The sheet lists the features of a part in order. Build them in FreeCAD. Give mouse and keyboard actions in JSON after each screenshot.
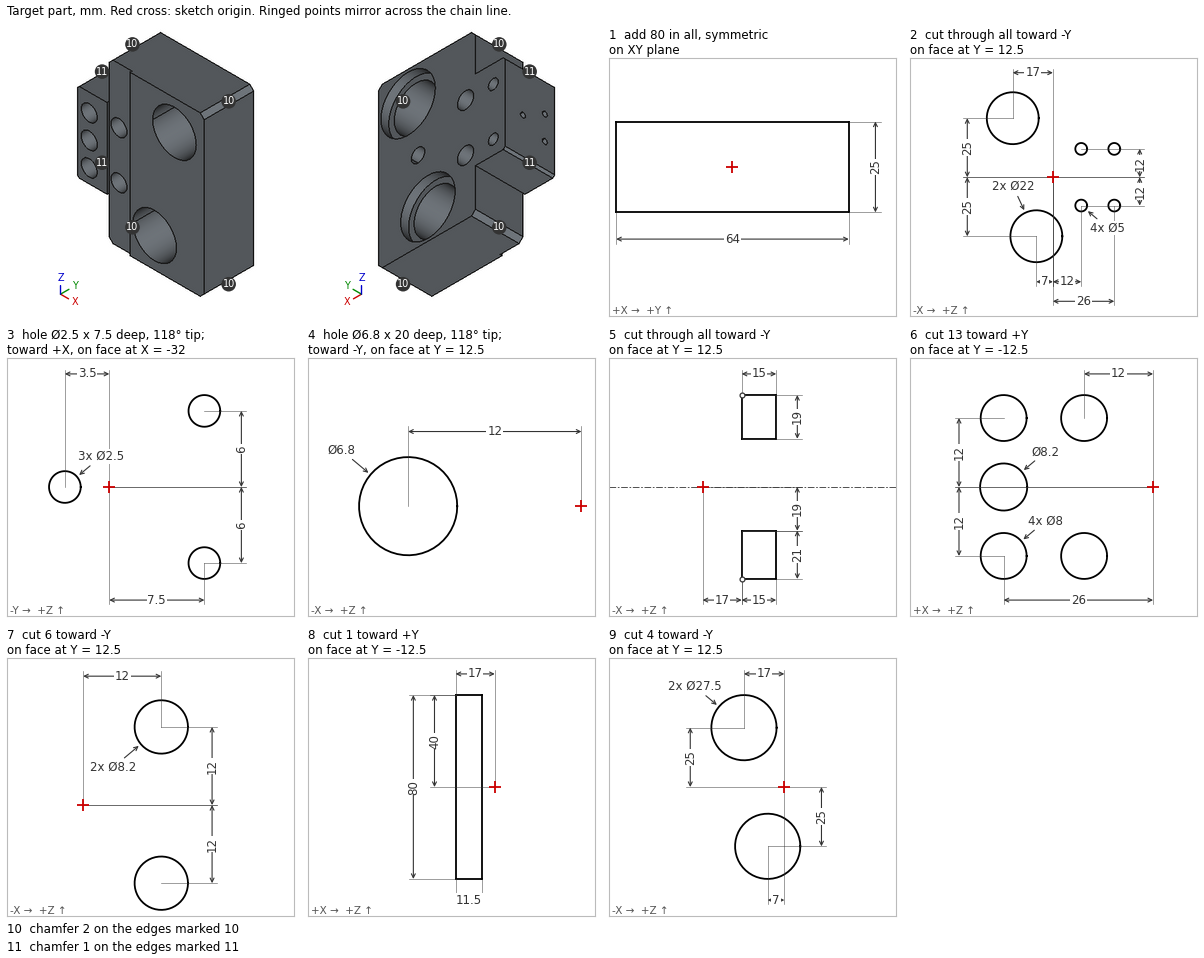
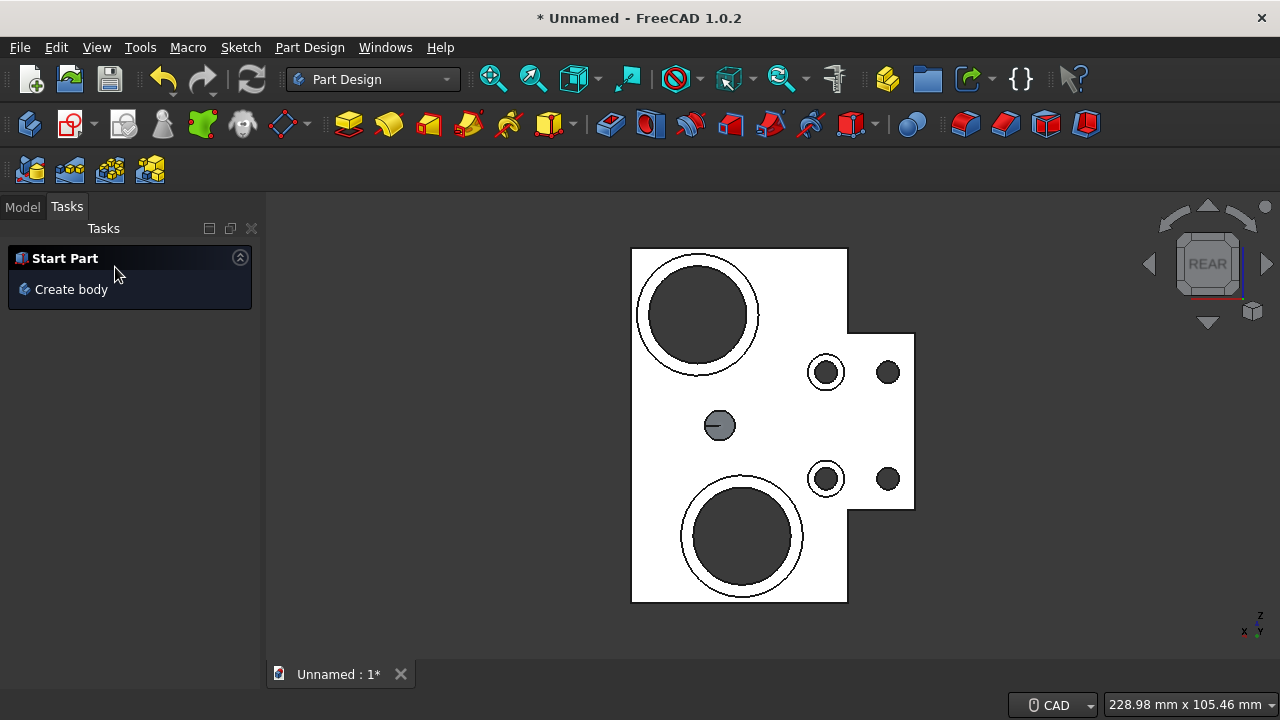
{"action": "key", "text": "0"}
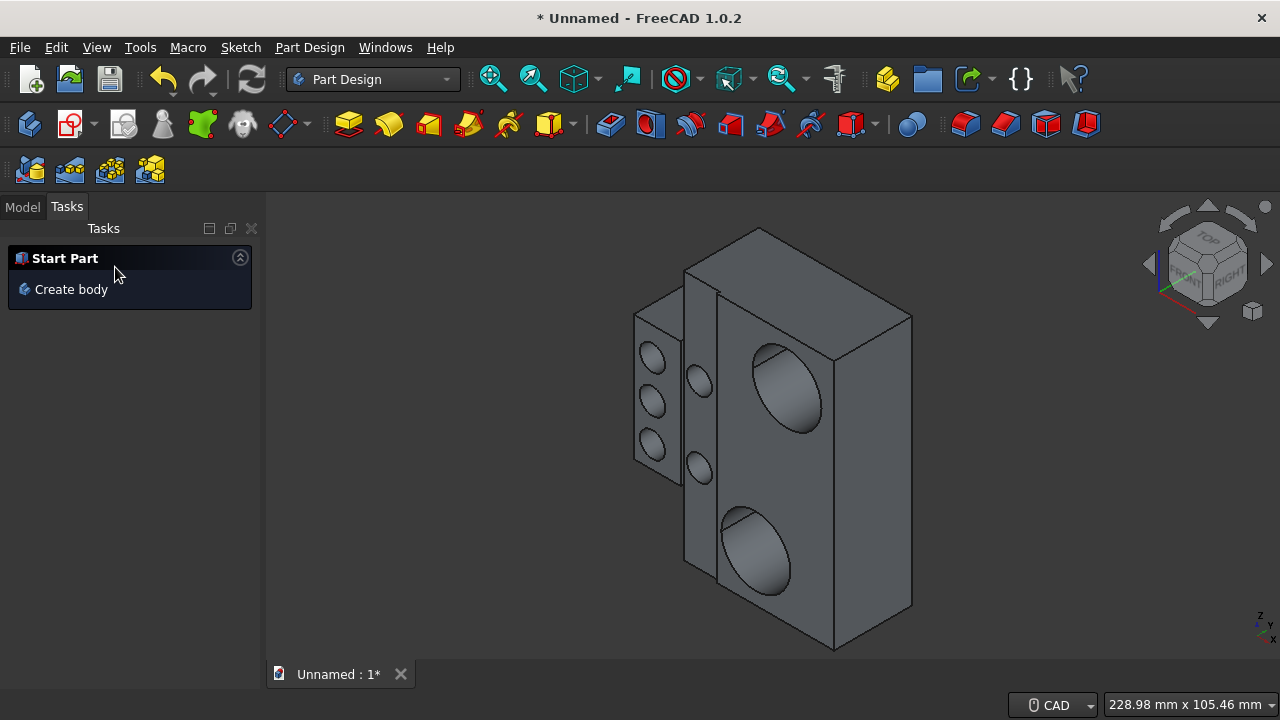
{"action": "left_click", "coordinate": [873, 338]}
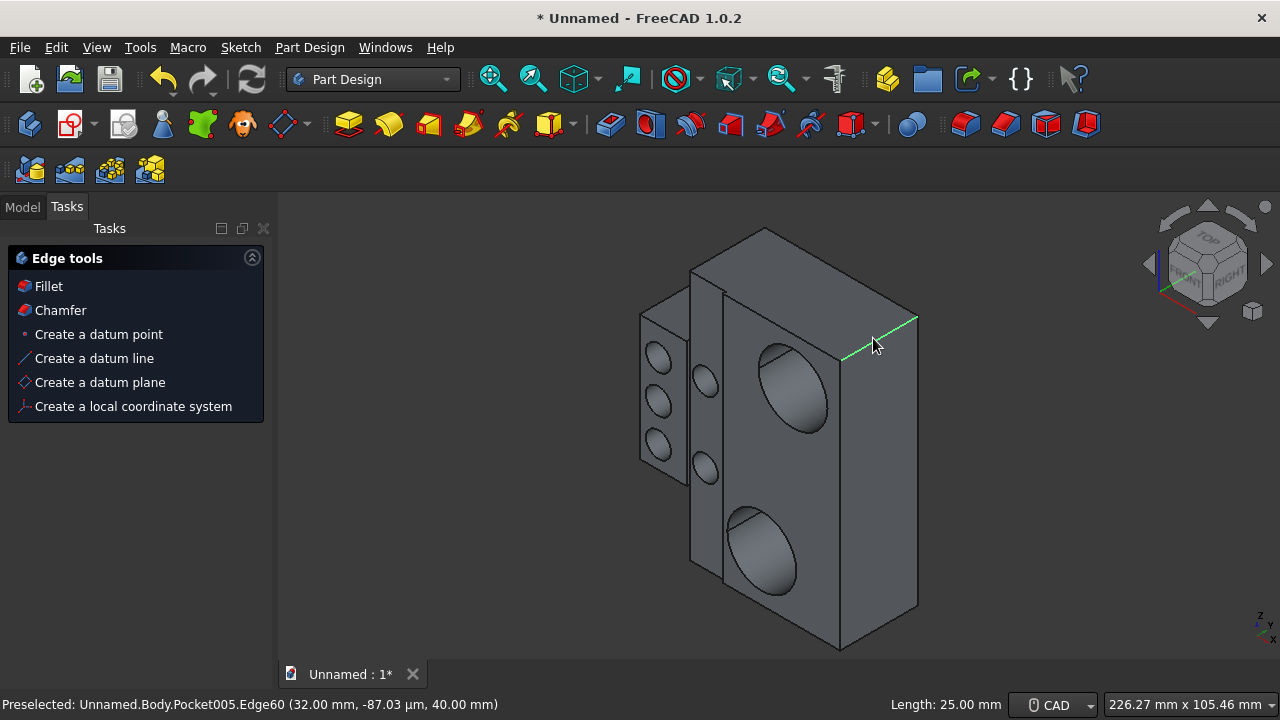
{"action": "key", "text": "2"}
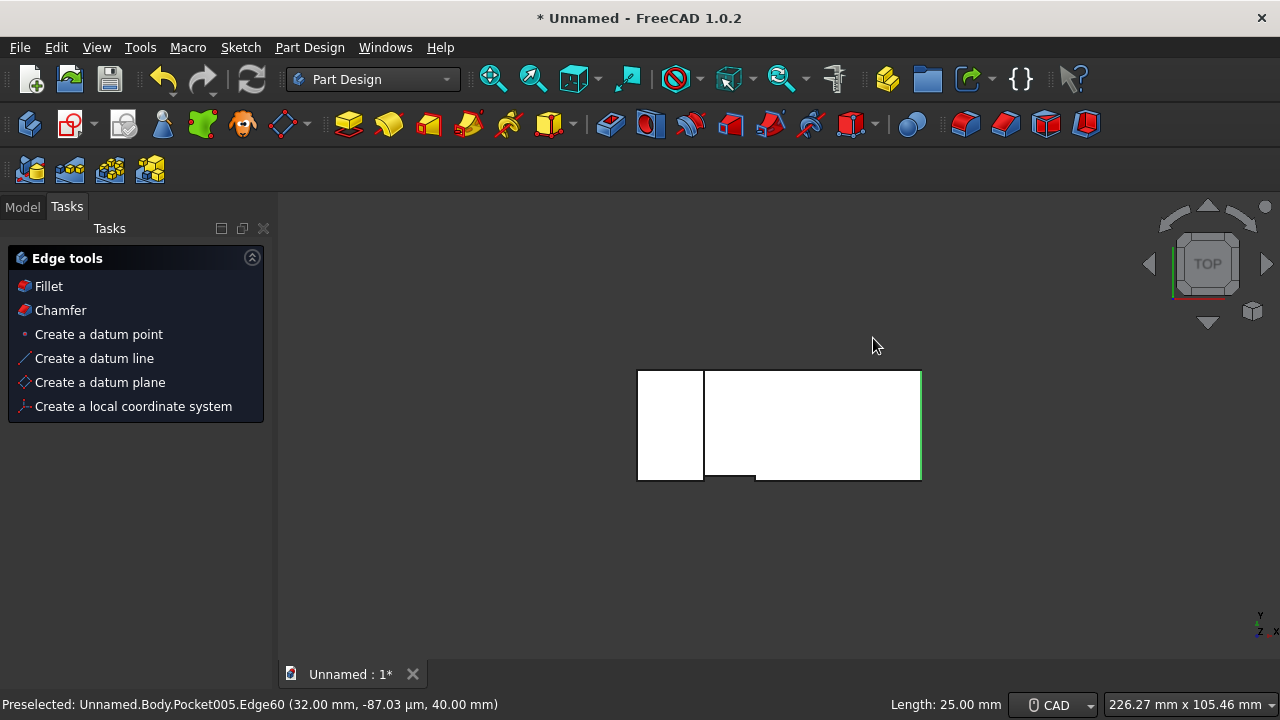
{"action": "left_click", "coordinate": [494, 80]}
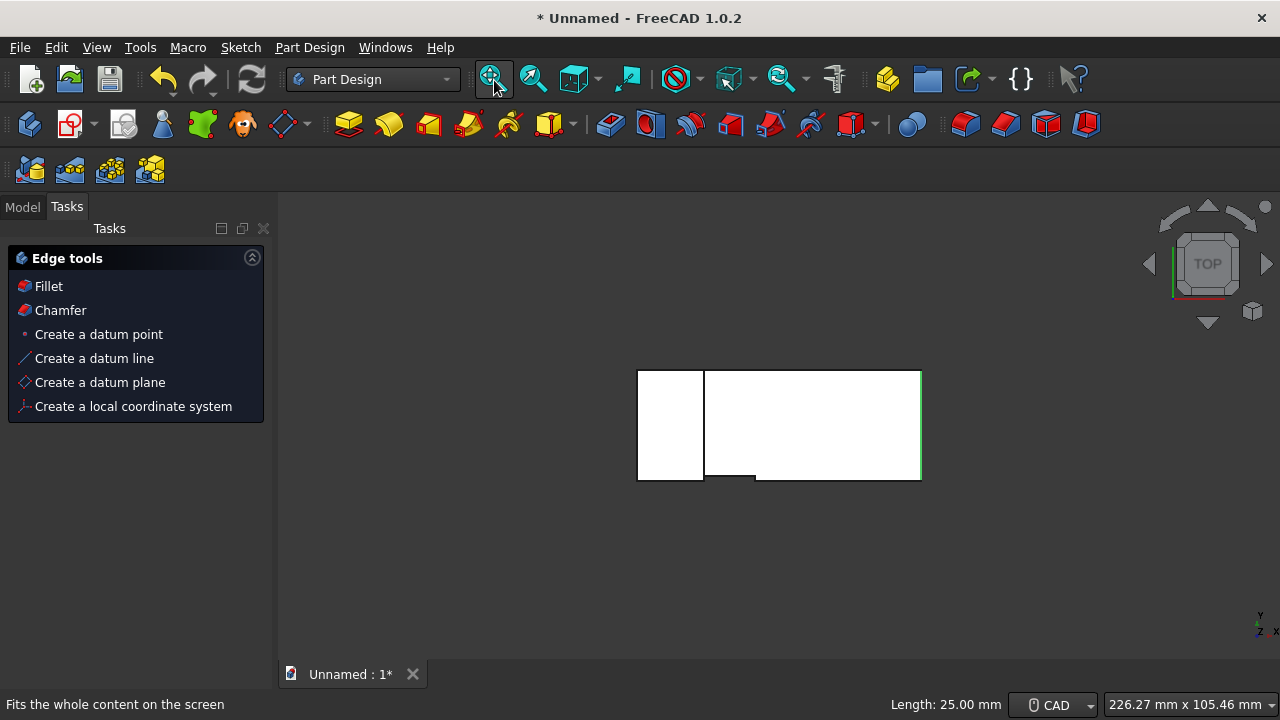
{"action": "left_click", "coordinate": [704, 422], "text": "ctrl"}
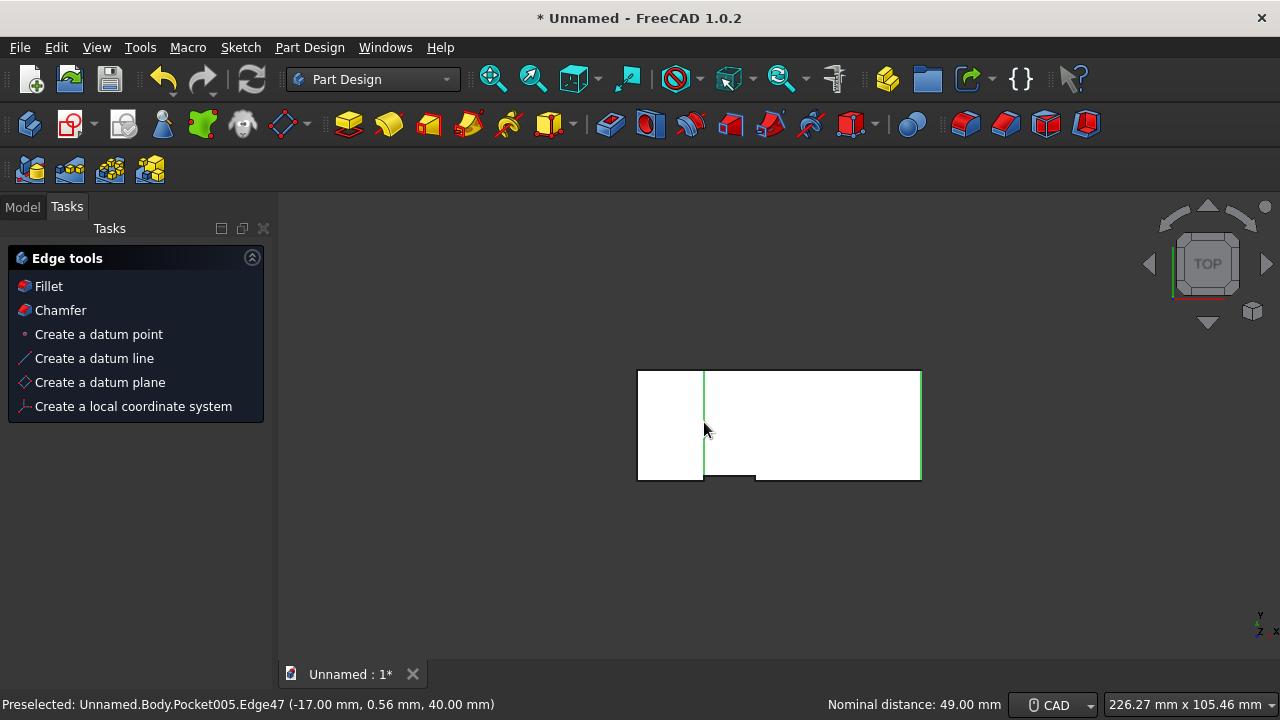
{"action": "key", "text": "1"}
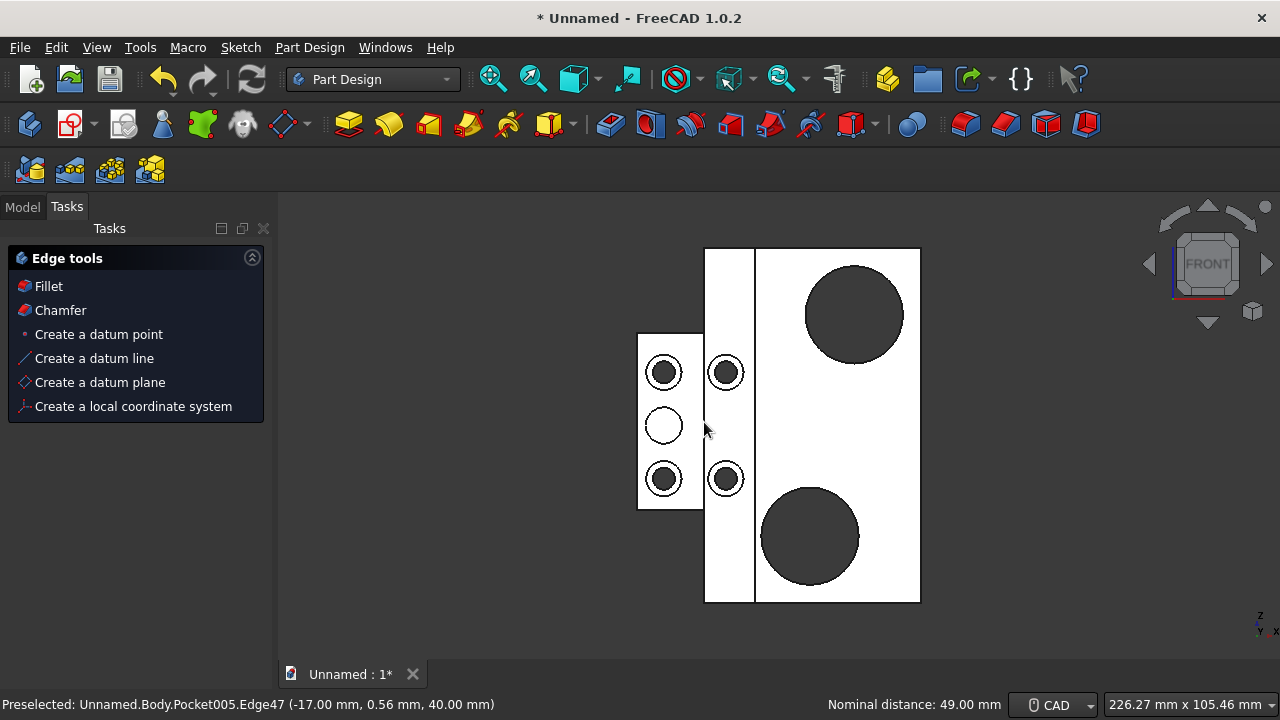
{"action": "key", "text": "3"}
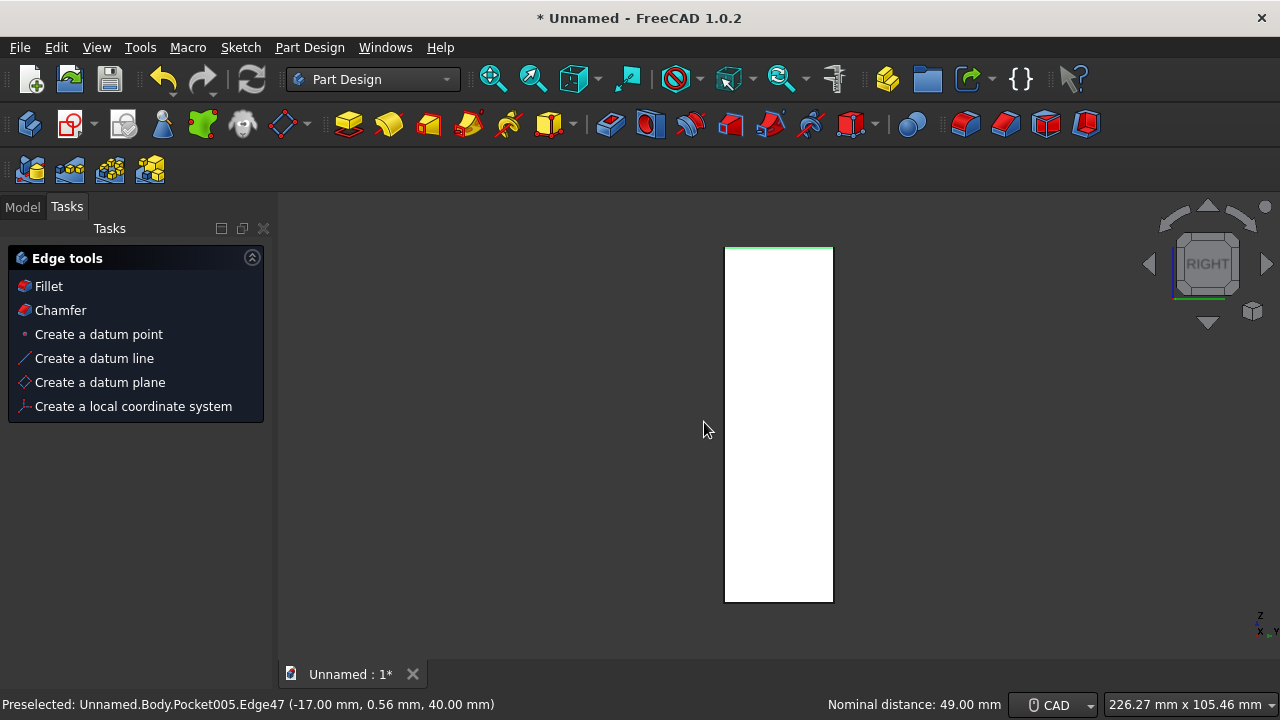
{"action": "left_click", "coordinate": [779, 602], "text": "ctrl"}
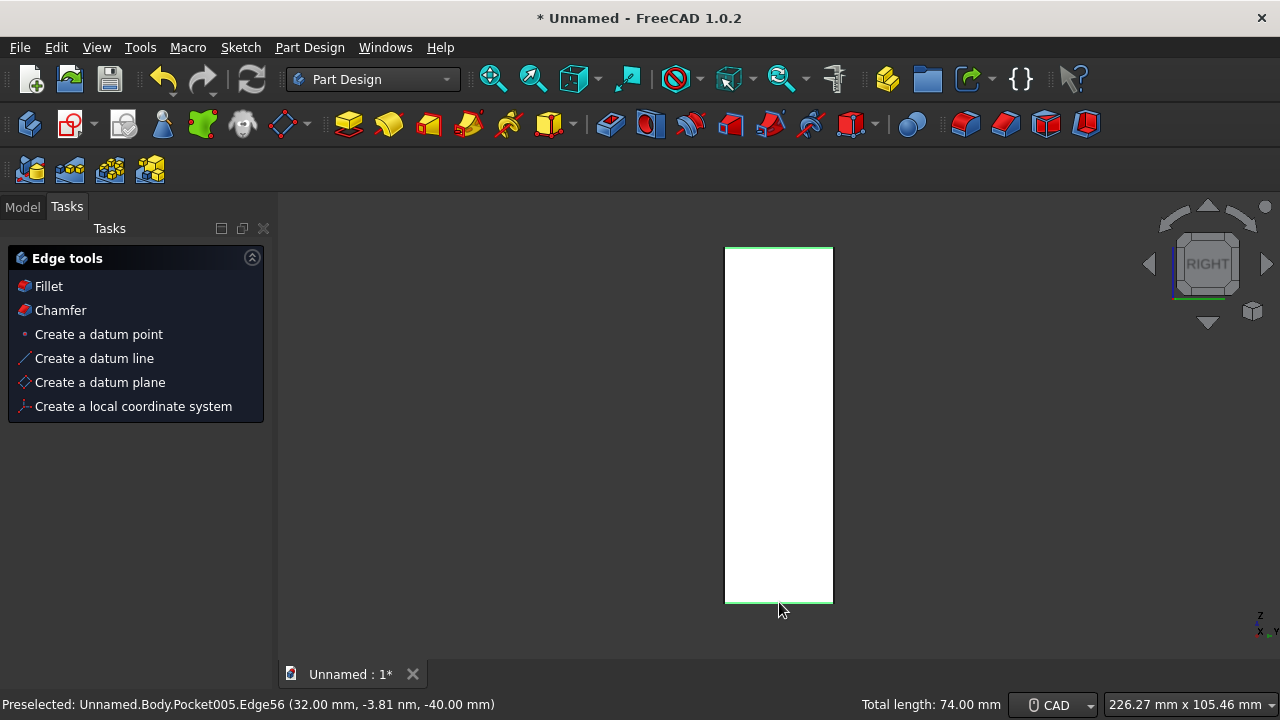
{"action": "key", "text": "5"}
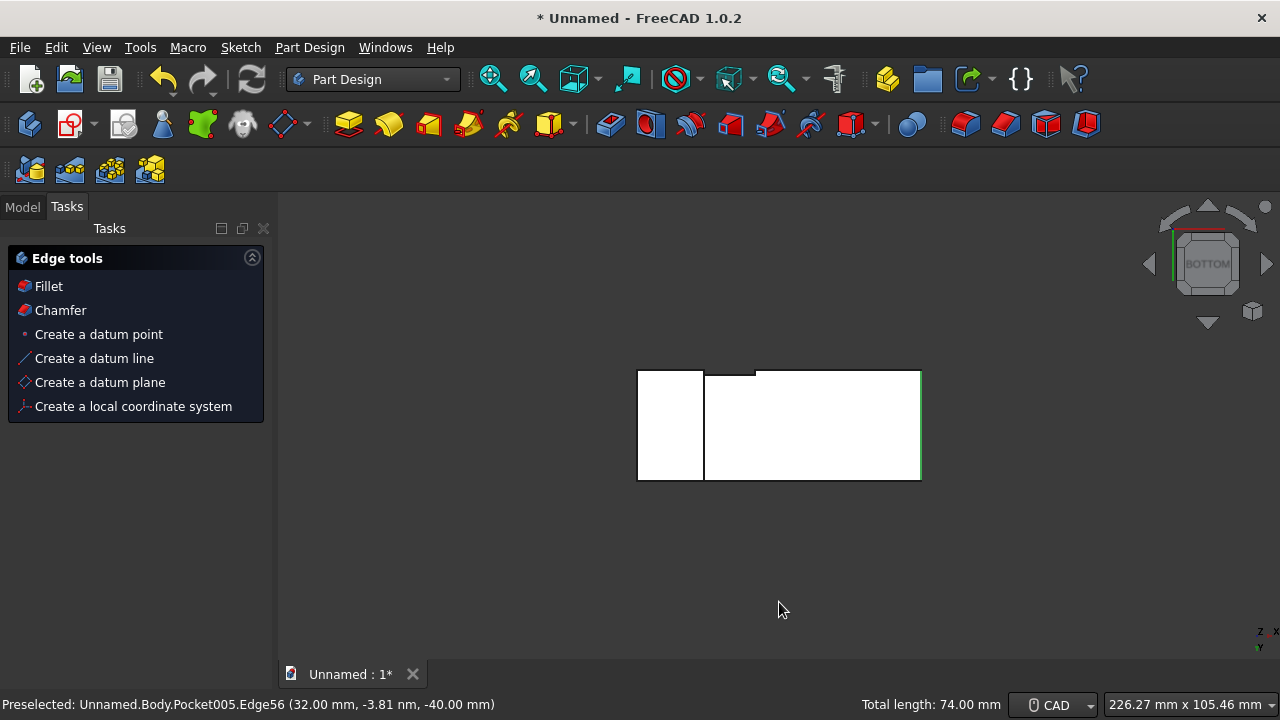
{"action": "left_click", "coordinate": [494, 80]}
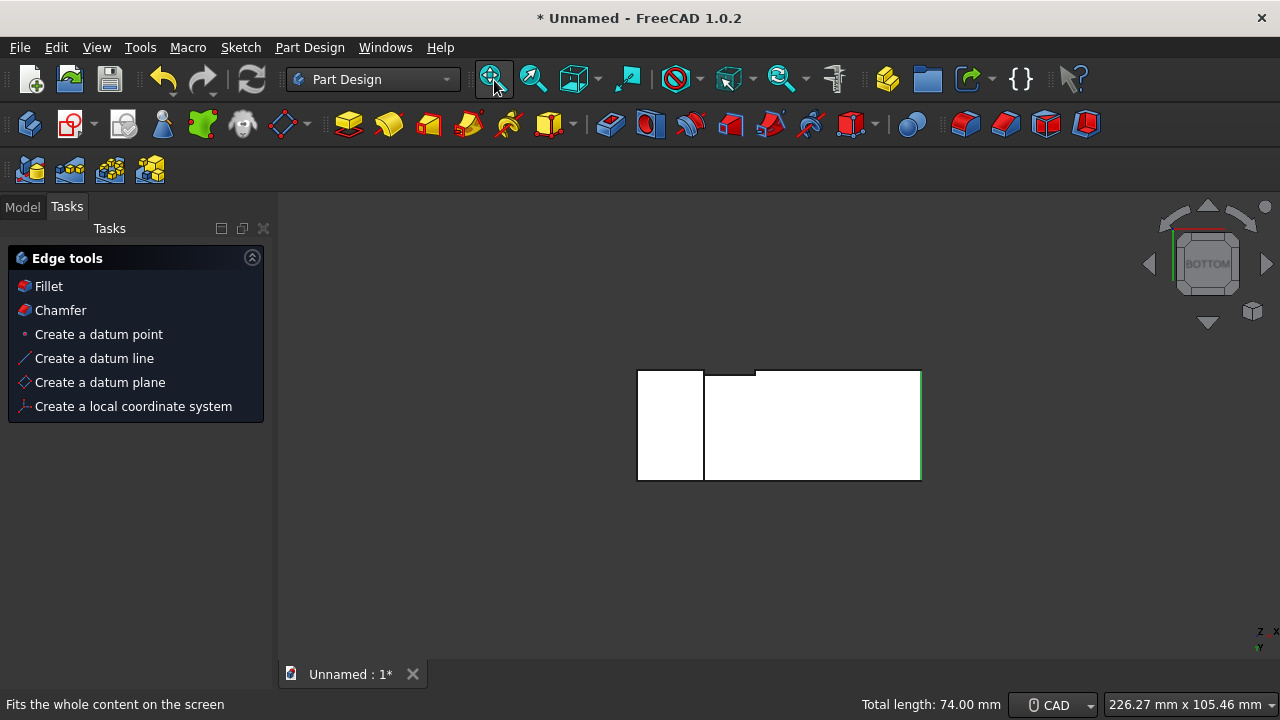
{"action": "left_click", "coordinate": [704, 427], "text": "ctrl"}